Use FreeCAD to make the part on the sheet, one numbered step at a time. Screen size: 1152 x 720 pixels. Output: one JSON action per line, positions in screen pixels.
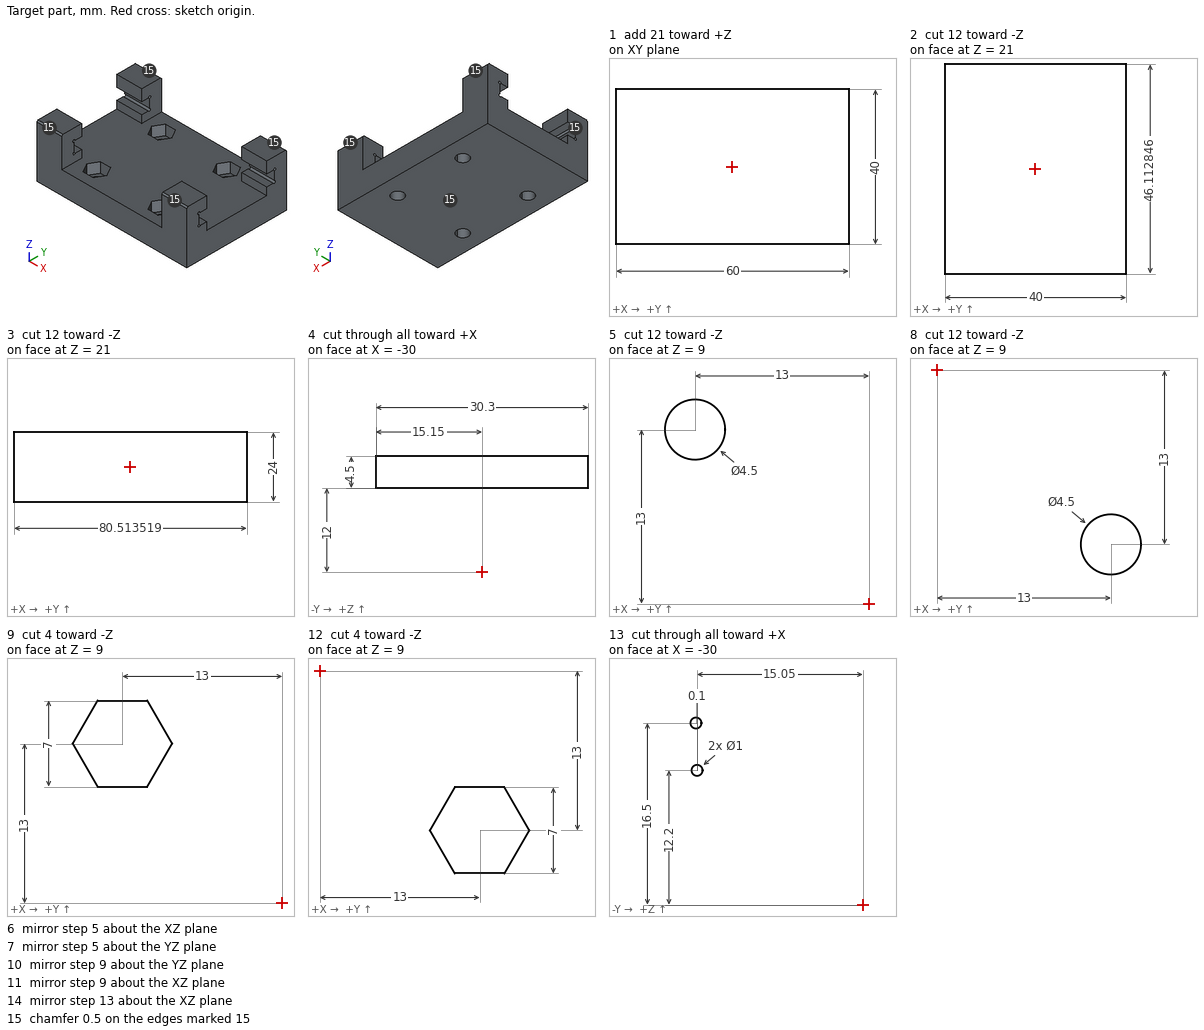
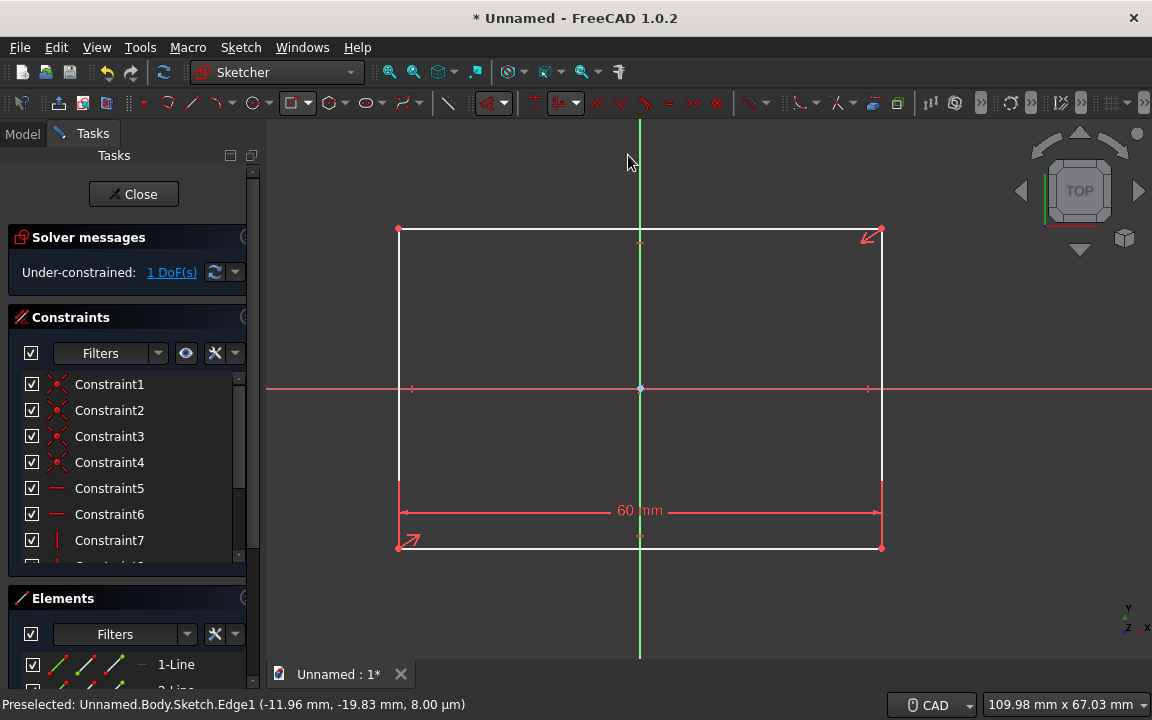
{"action": "left_click", "coordinate": [882, 453]}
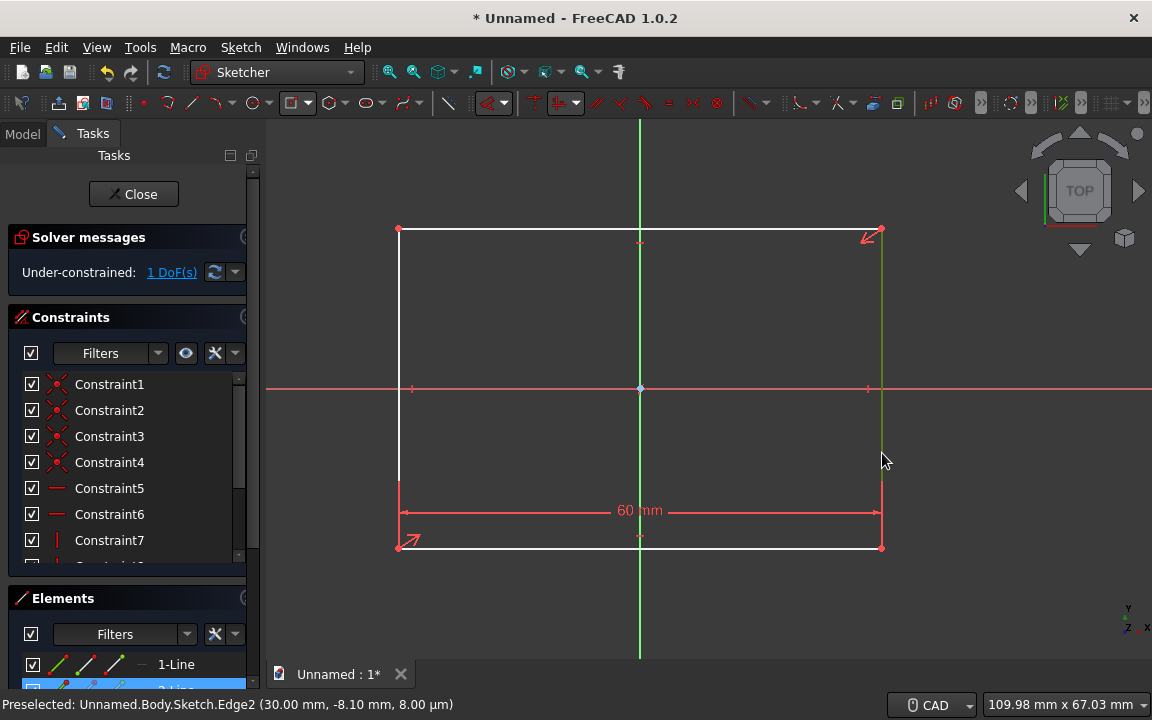
{"action": "left_click", "coordinate": [506, 104]}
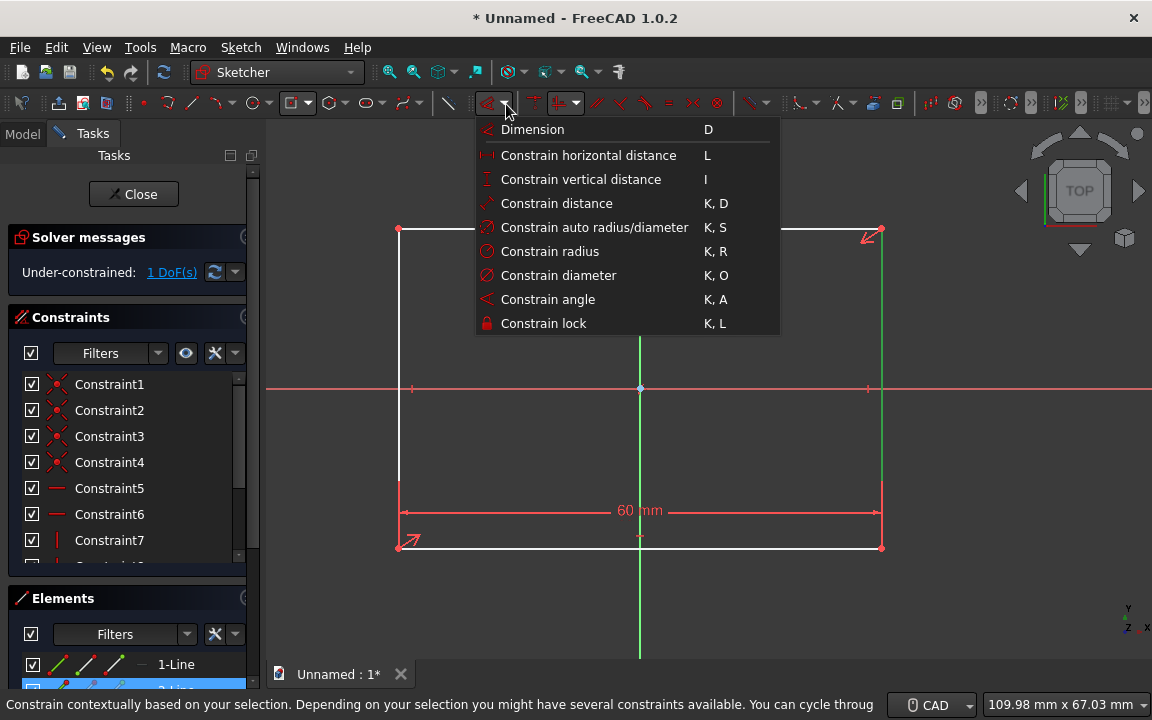
{"action": "left_click", "coordinate": [628, 179]}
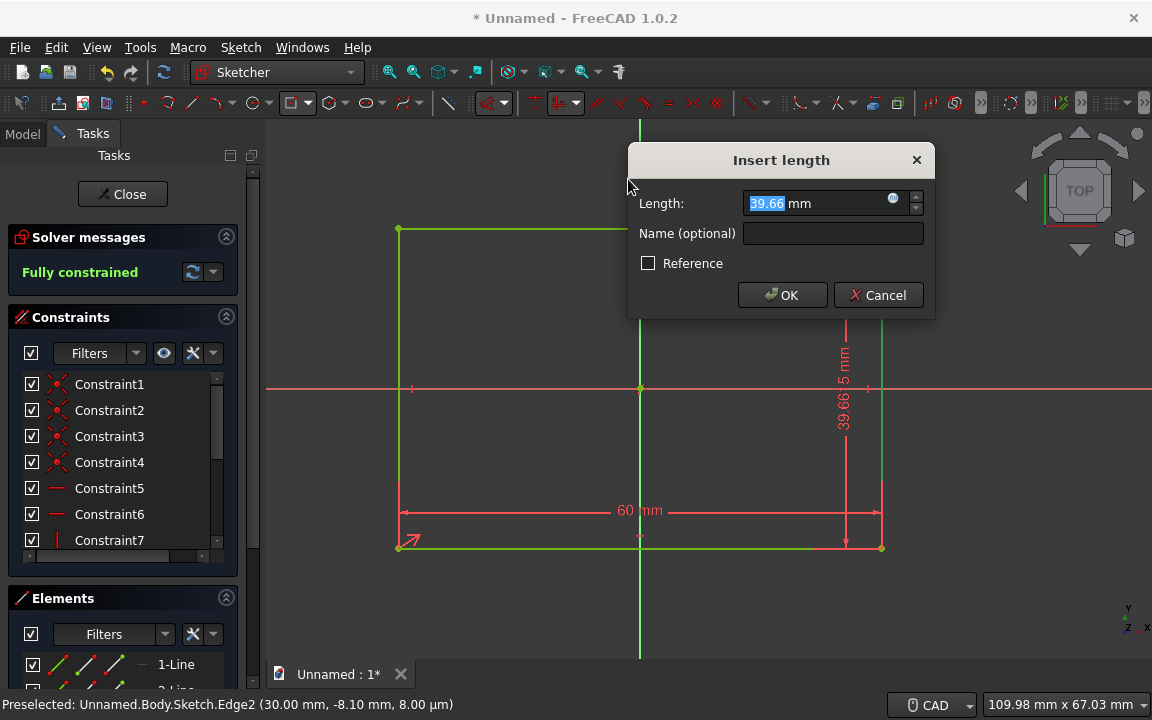
{"action": "type", "text": "40"}
{"action": "key", "text": "Return"}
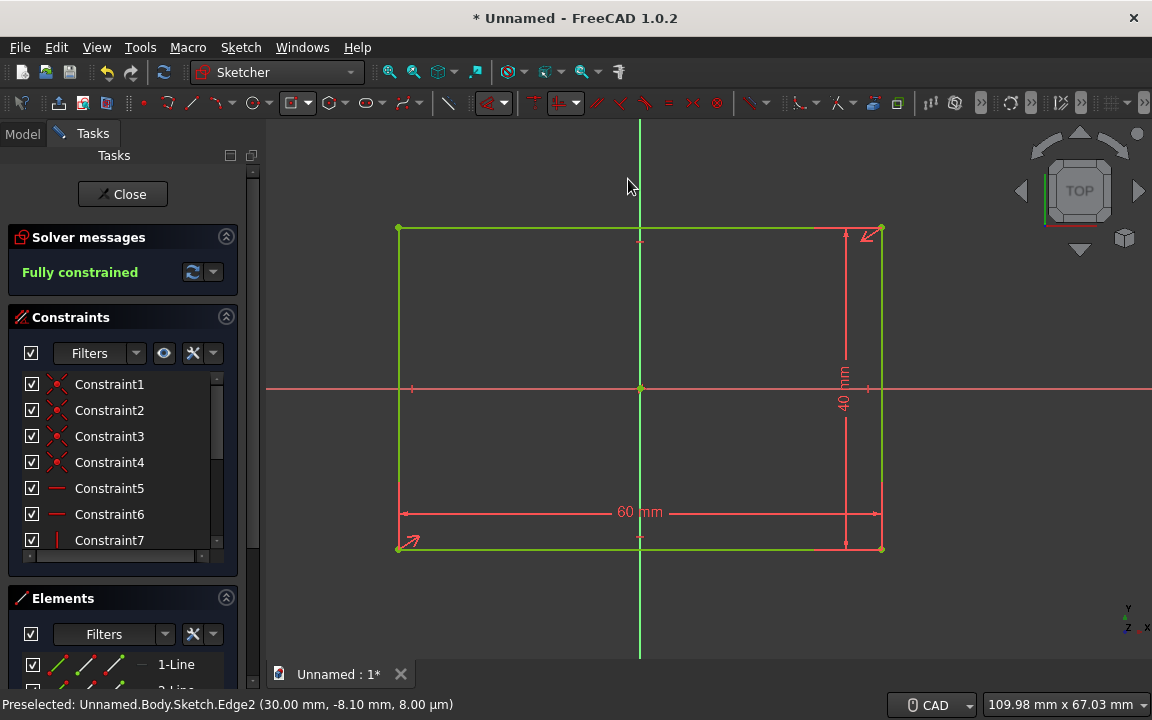
{"action": "left_click", "coordinate": [123, 194]}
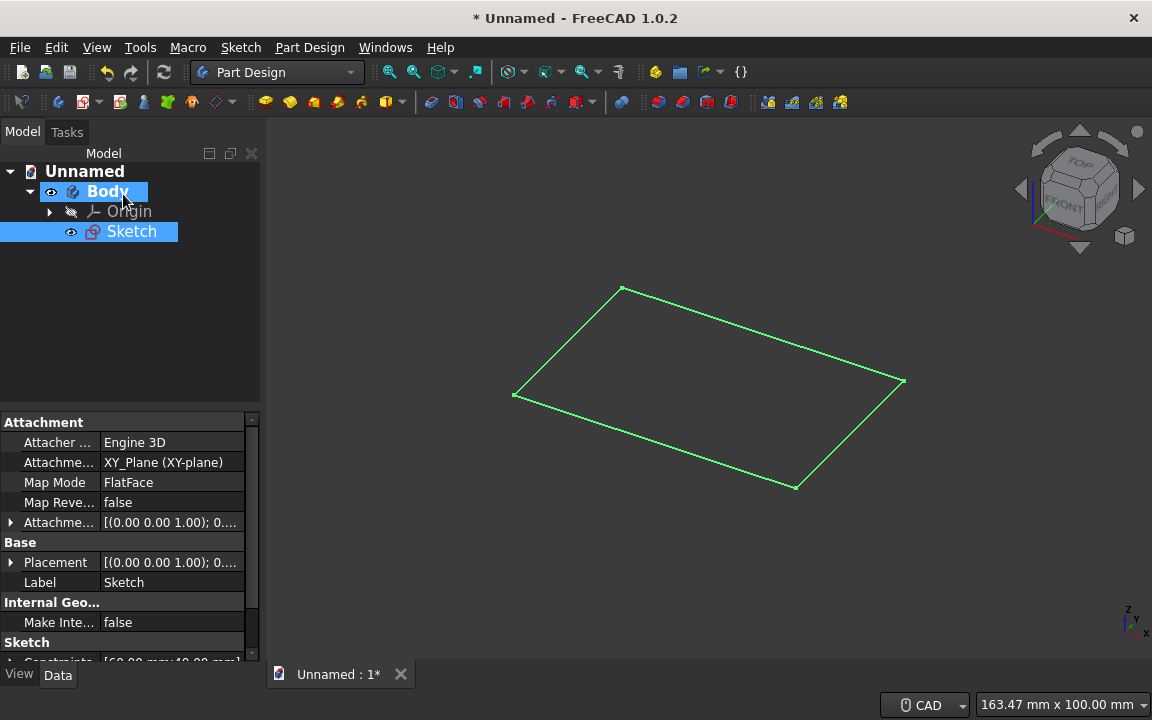
{"action": "left_click", "coordinate": [266, 102]}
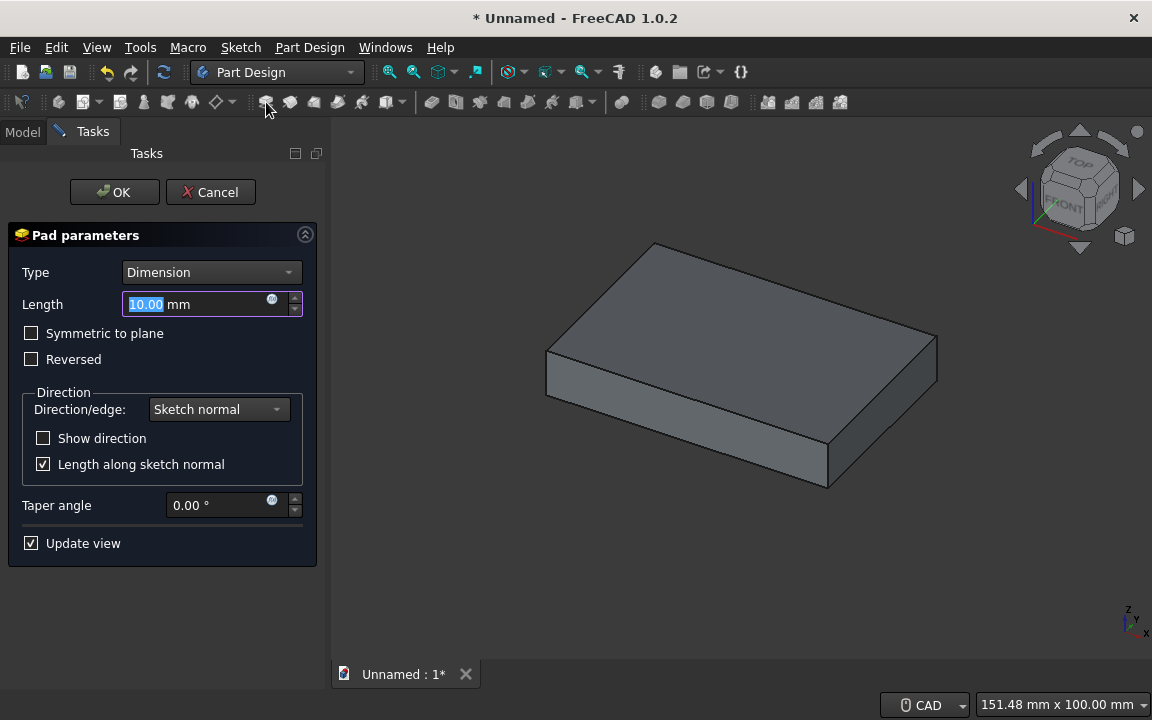
{"action": "type", "text": "21"}
{"action": "key", "text": "Tab"}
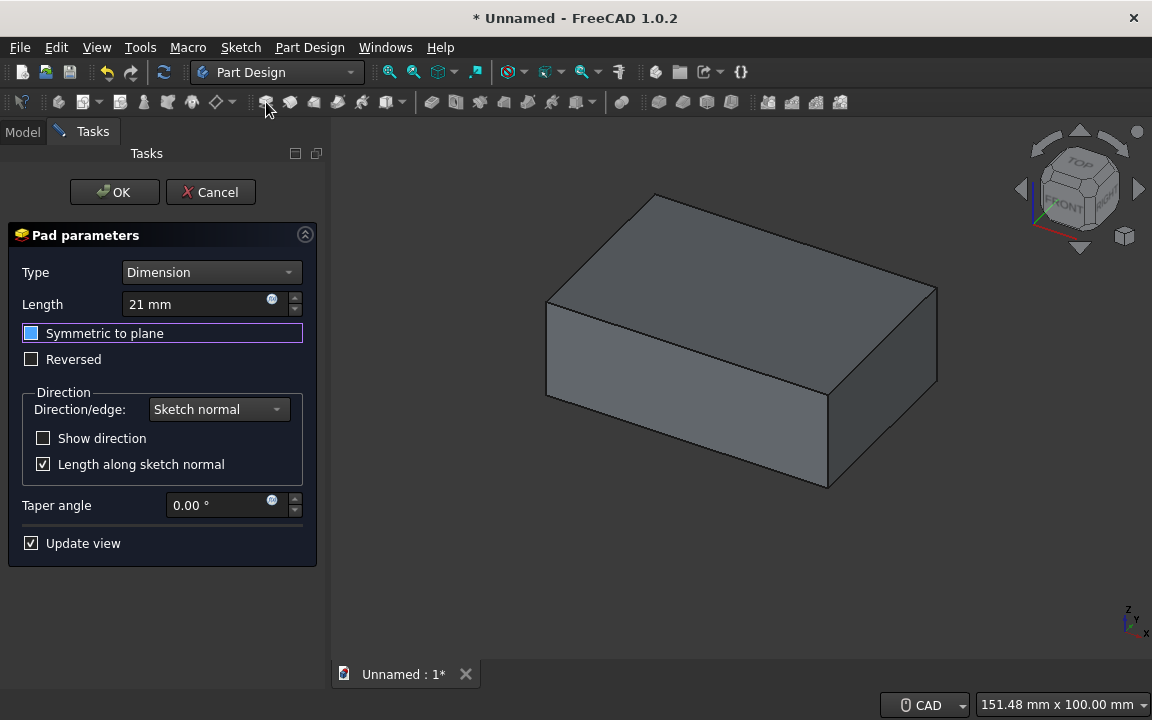
{"action": "left_click", "coordinate": [115, 192]}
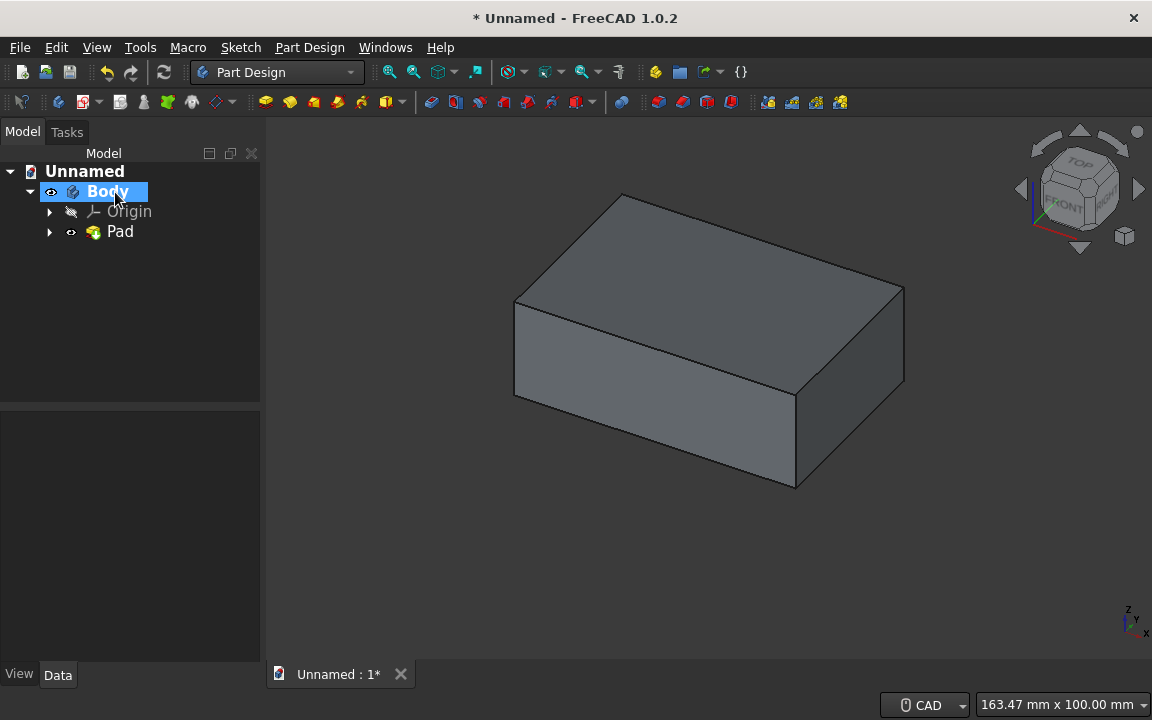
{"action": "left_click", "coordinate": [749, 307]}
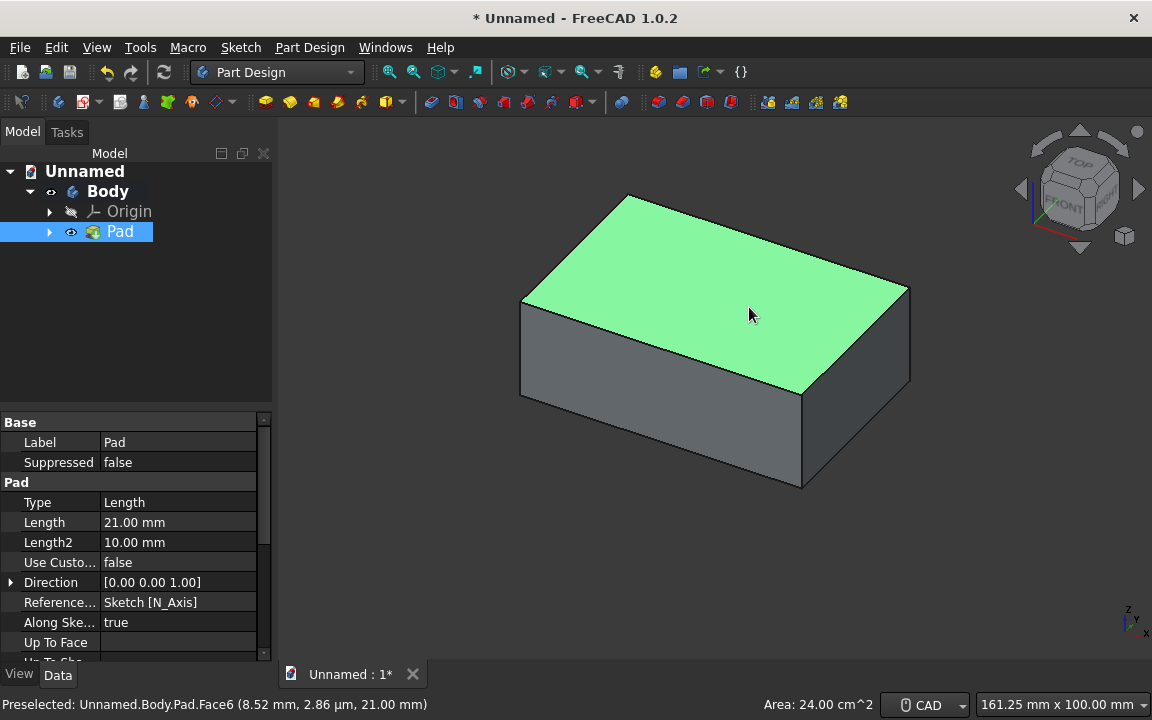
{"action": "left_click", "coordinate": [84, 102]}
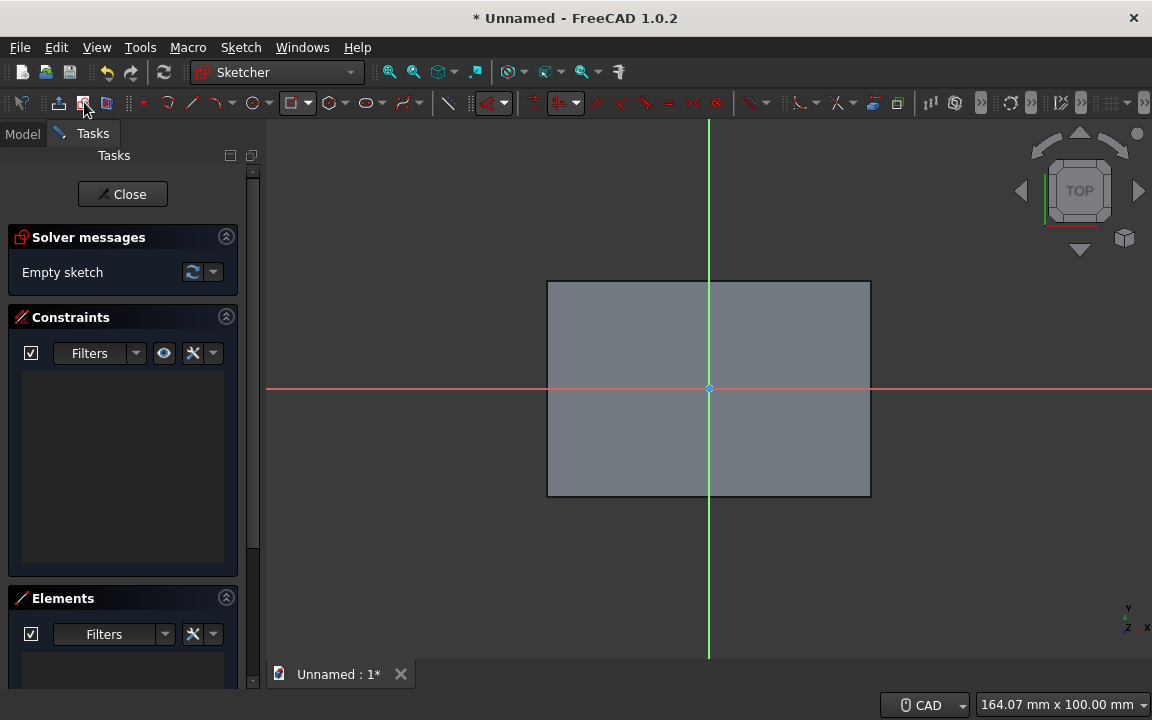
{"action": "scroll", "coordinate": [848, 389], "scroll_direction": "up", "scroll_amount": 2}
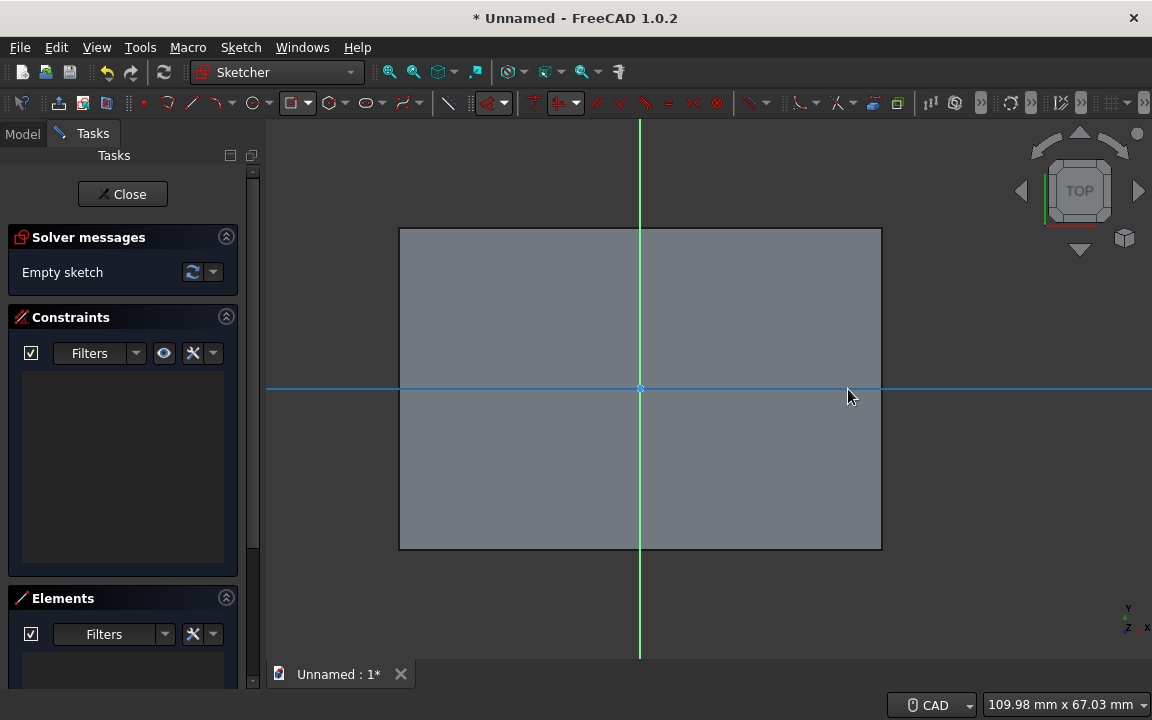
{"action": "left_click", "coordinate": [292, 104]}